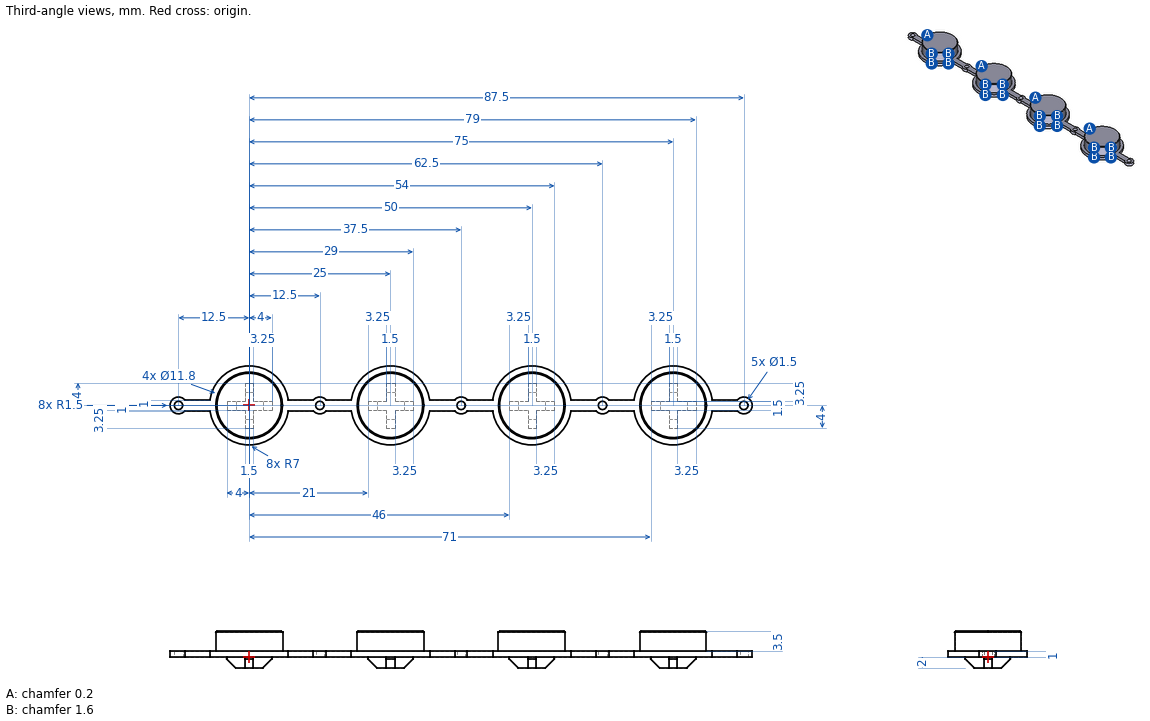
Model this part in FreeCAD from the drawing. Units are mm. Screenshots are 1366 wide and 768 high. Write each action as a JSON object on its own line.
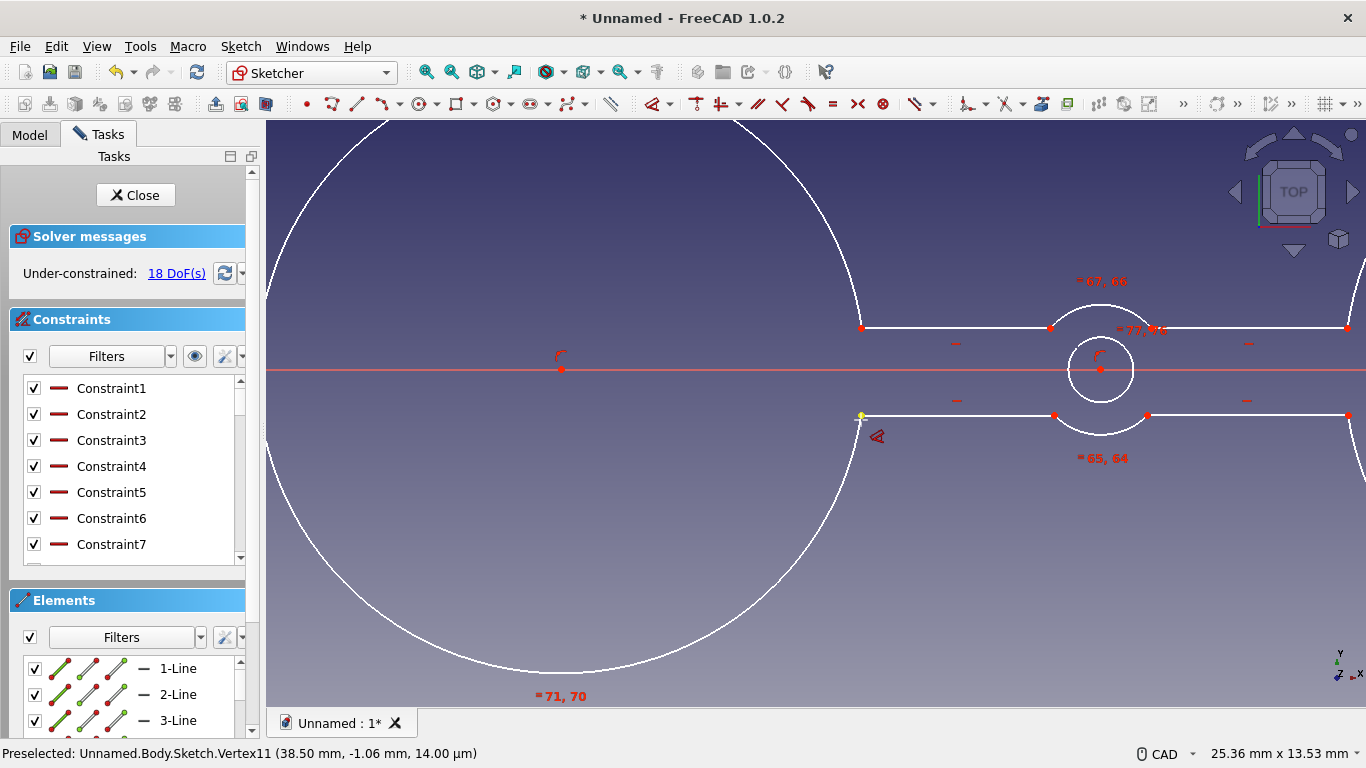
{"action": "left_click", "coordinate": [861, 416]}
{"action": "left_click", "coordinate": [895, 393]}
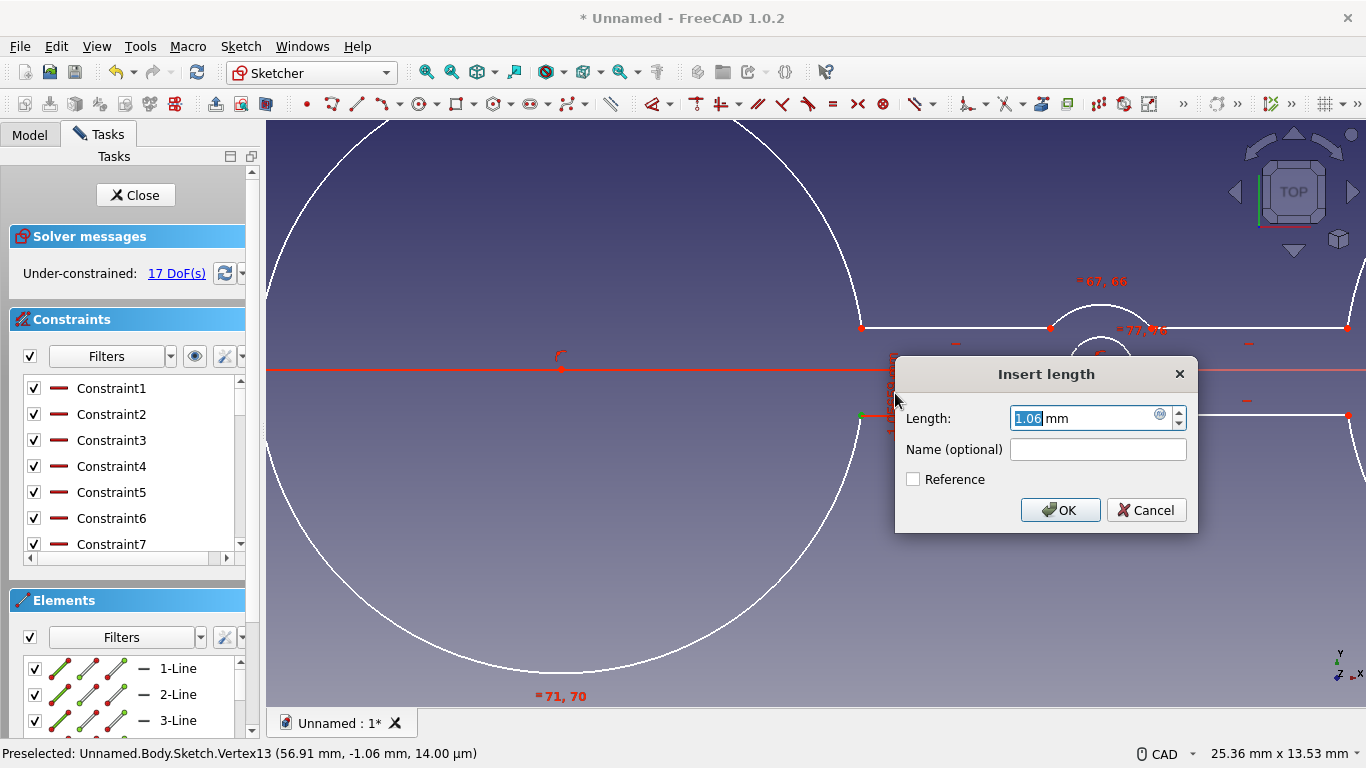
{"action": "type", "text": "1"}
{"action": "key", "text": "Return"}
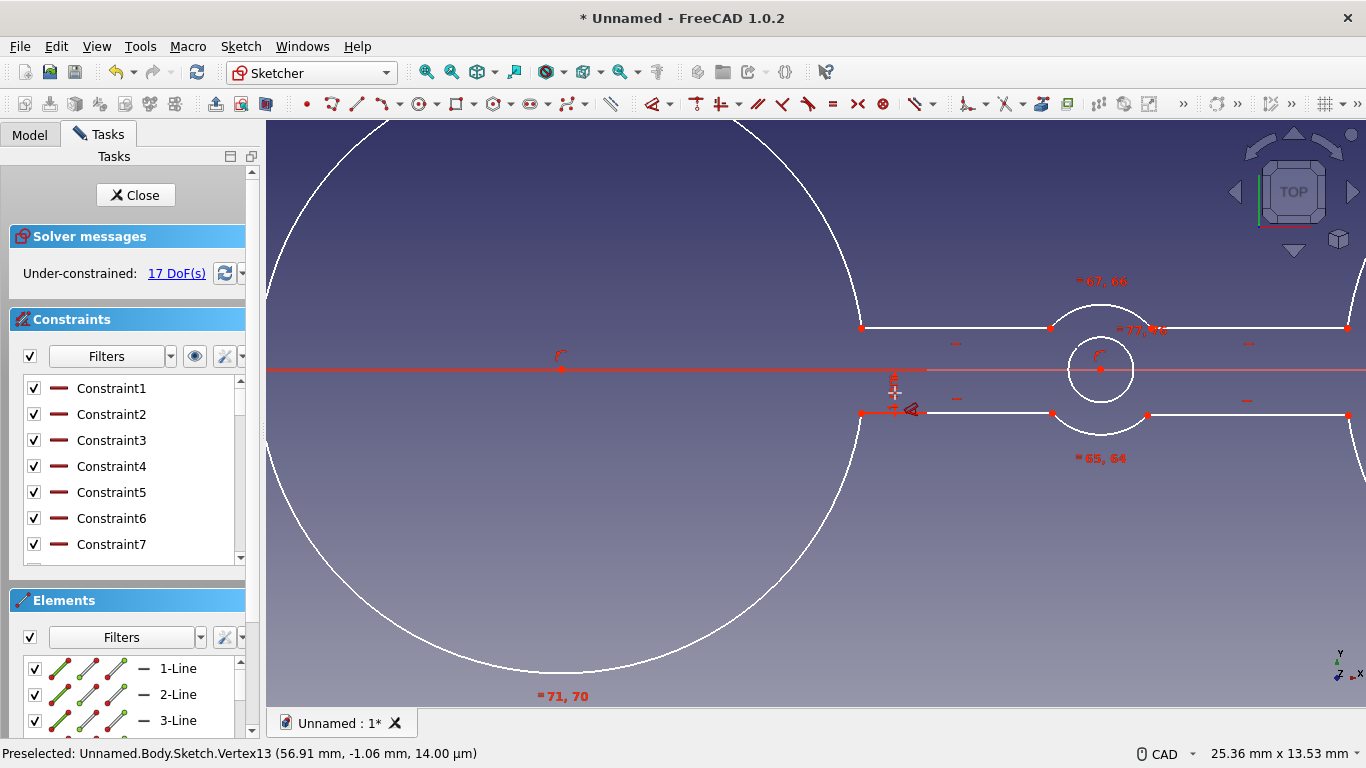
{"action": "left_click", "coordinate": [1148, 415]}
{"action": "left_click", "coordinate": [1182, 392]}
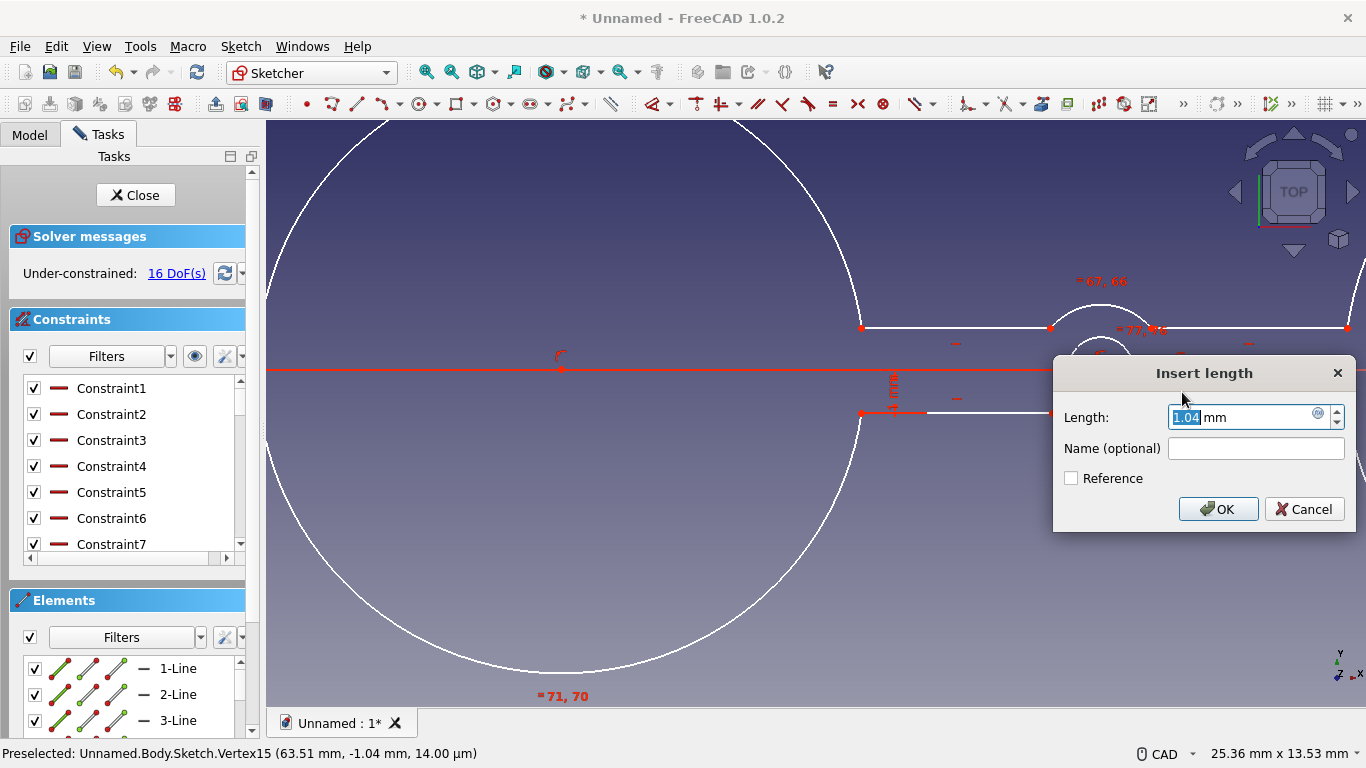
{"action": "type", "text": "1"}
{"action": "key", "text": "Return"}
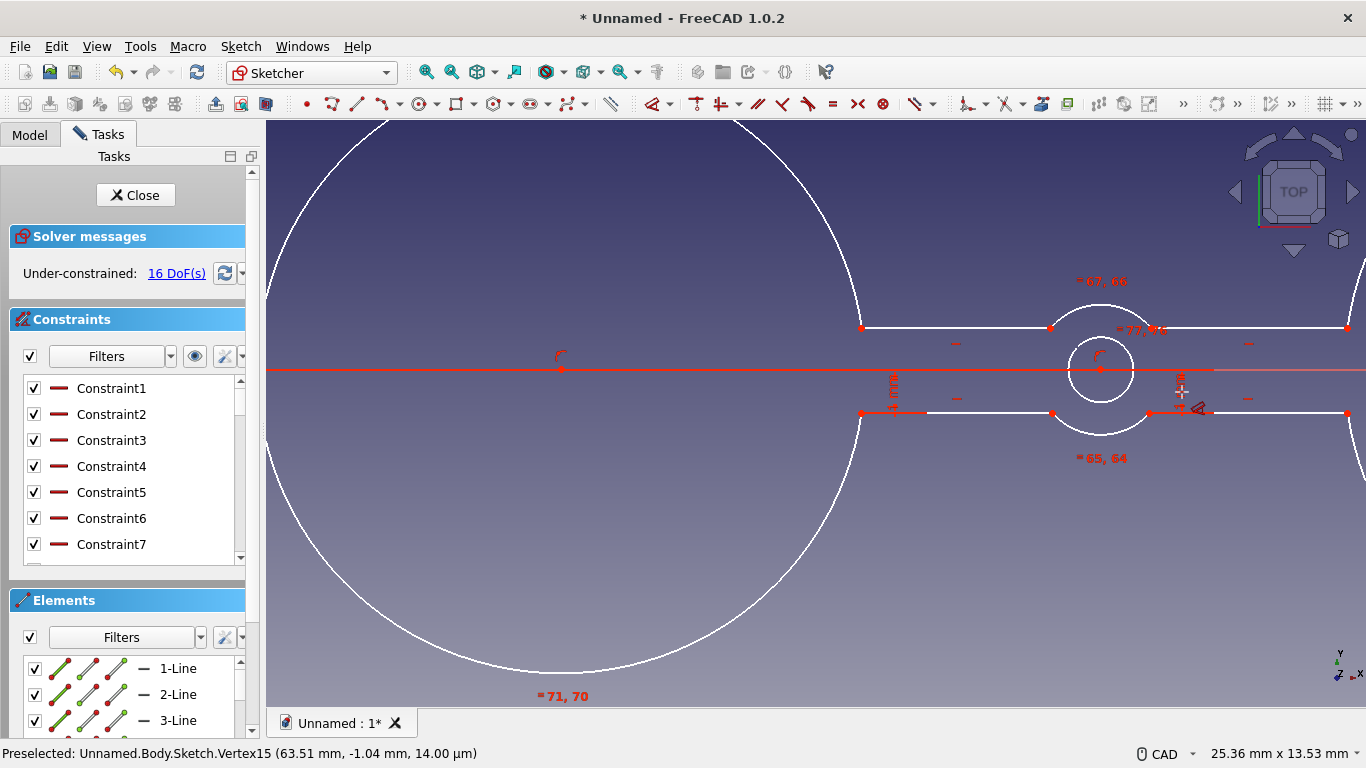
{"action": "scroll", "coordinate": [861, 420], "scroll_direction": "down", "scroll_amount": 10}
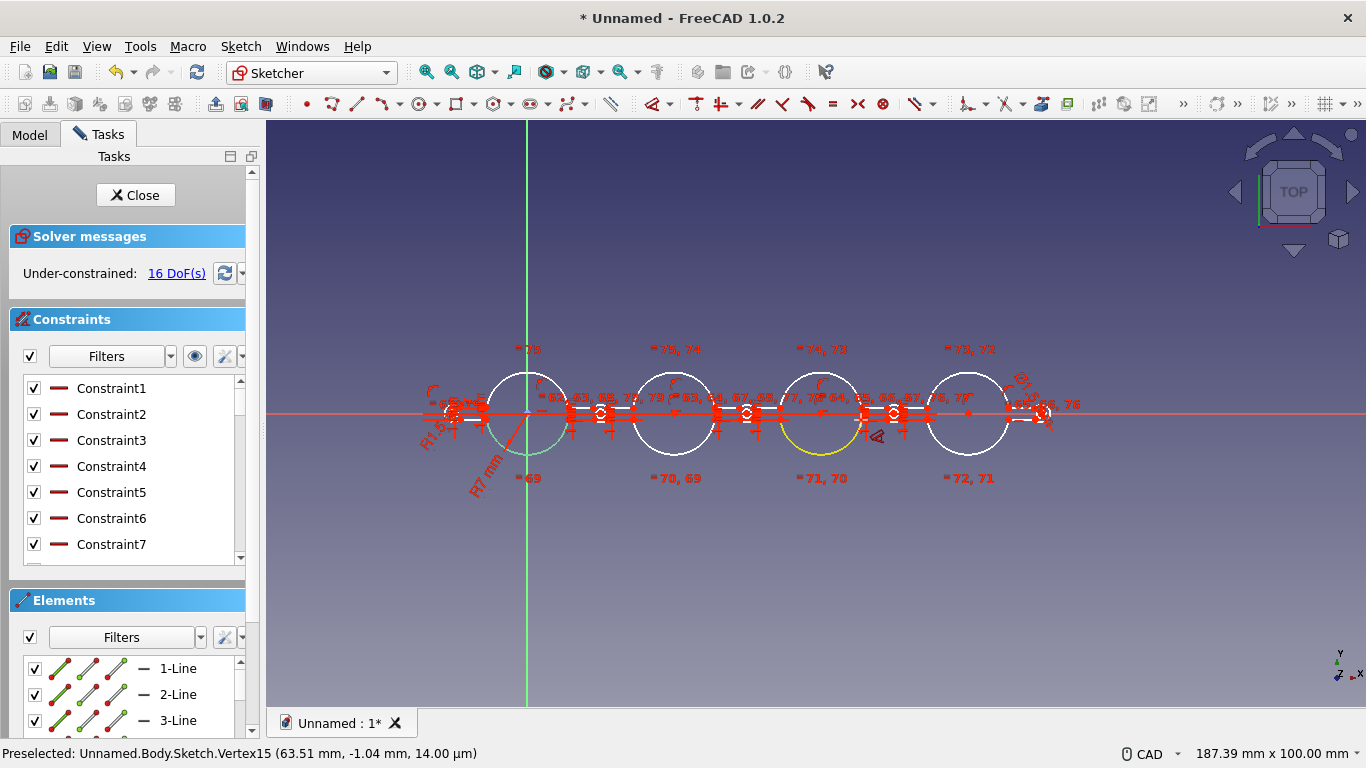
{"action": "scroll", "coordinate": [1009, 420], "scroll_direction": "up", "scroll_amount": 10}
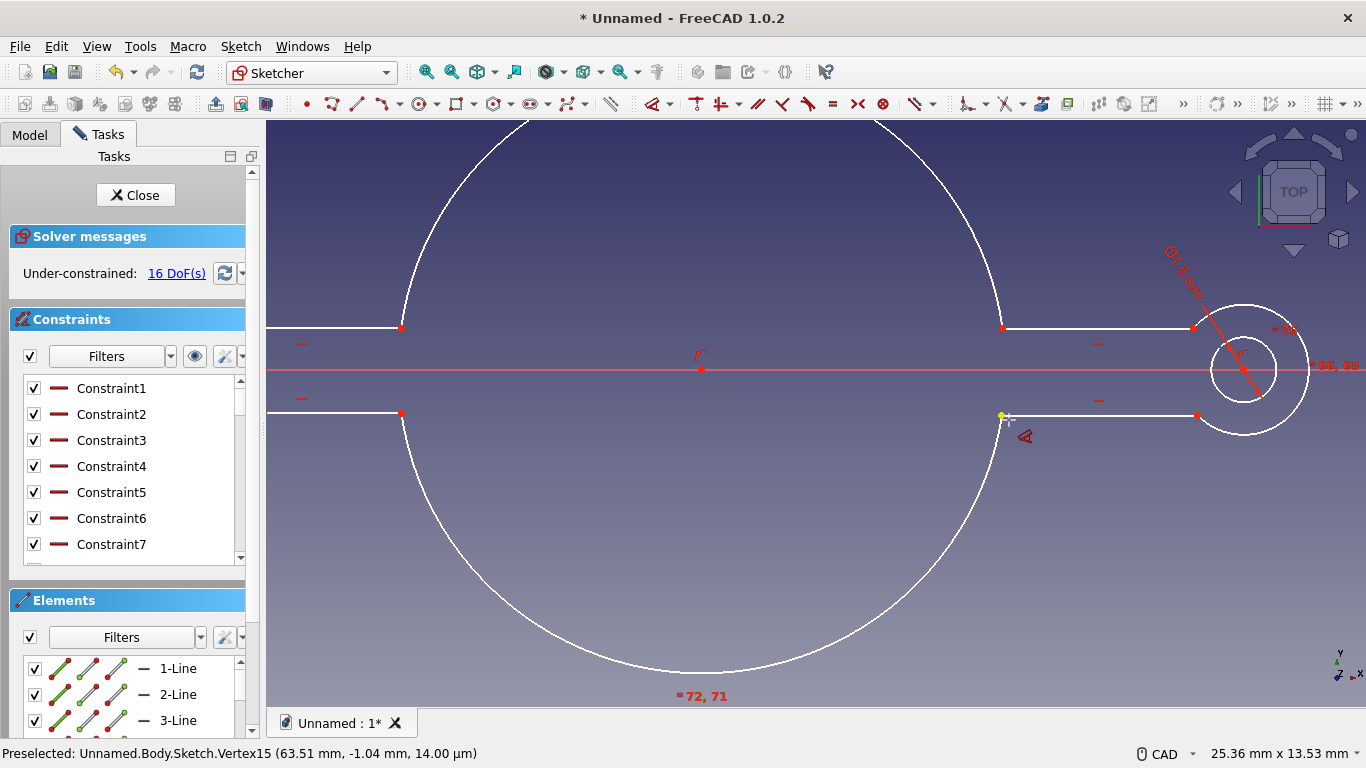
{"action": "left_click", "coordinate": [1002, 416]}
{"action": "left_click", "coordinate": [1036, 393]}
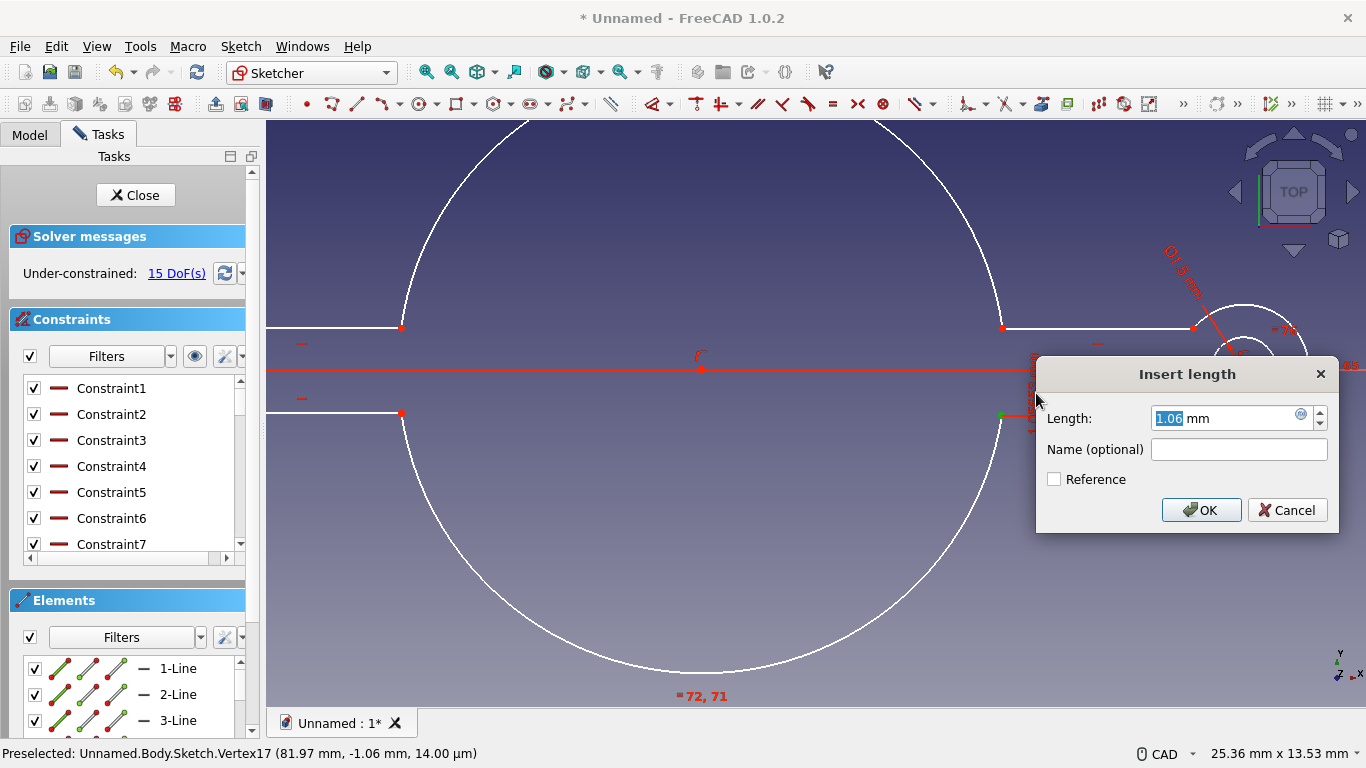
{"action": "type", "text": "1"}
{"action": "key", "text": "Return"}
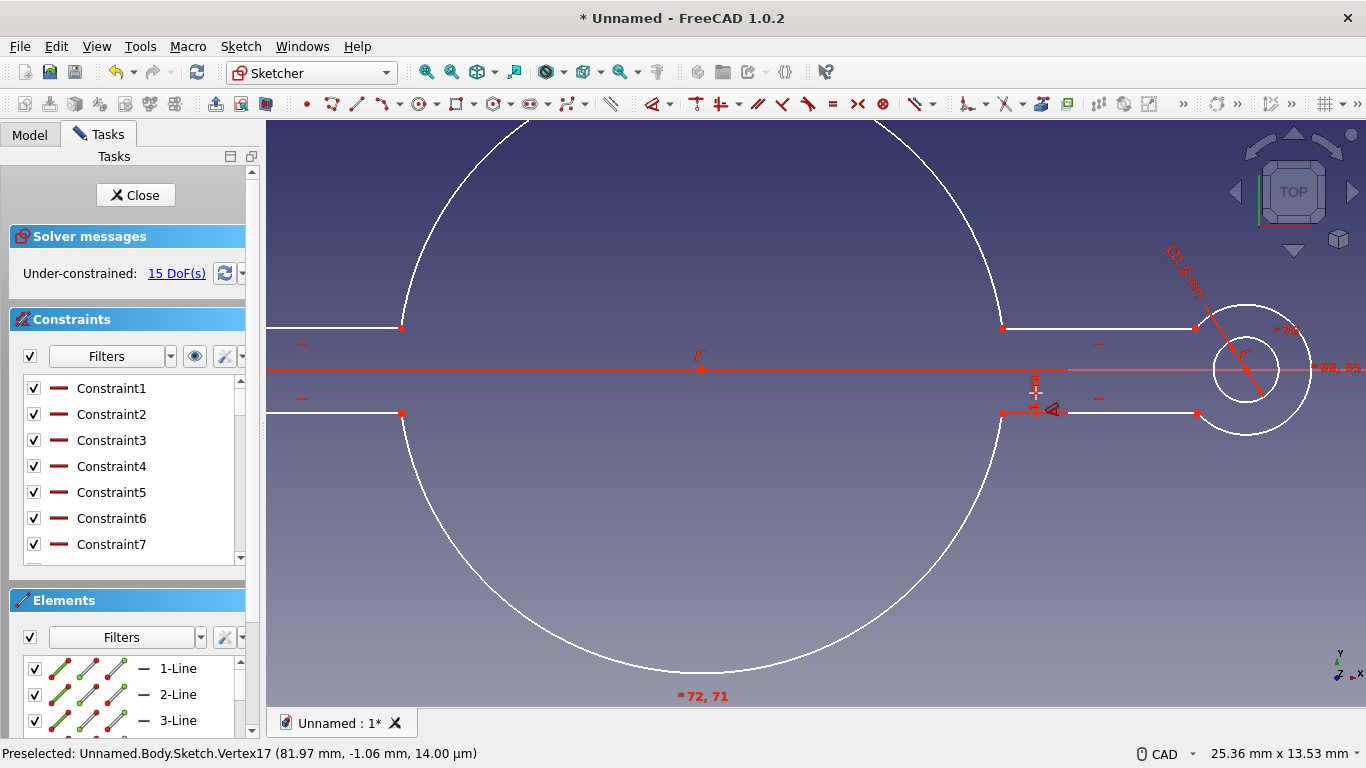
{"action": "left_click", "coordinate": [1196, 329]}